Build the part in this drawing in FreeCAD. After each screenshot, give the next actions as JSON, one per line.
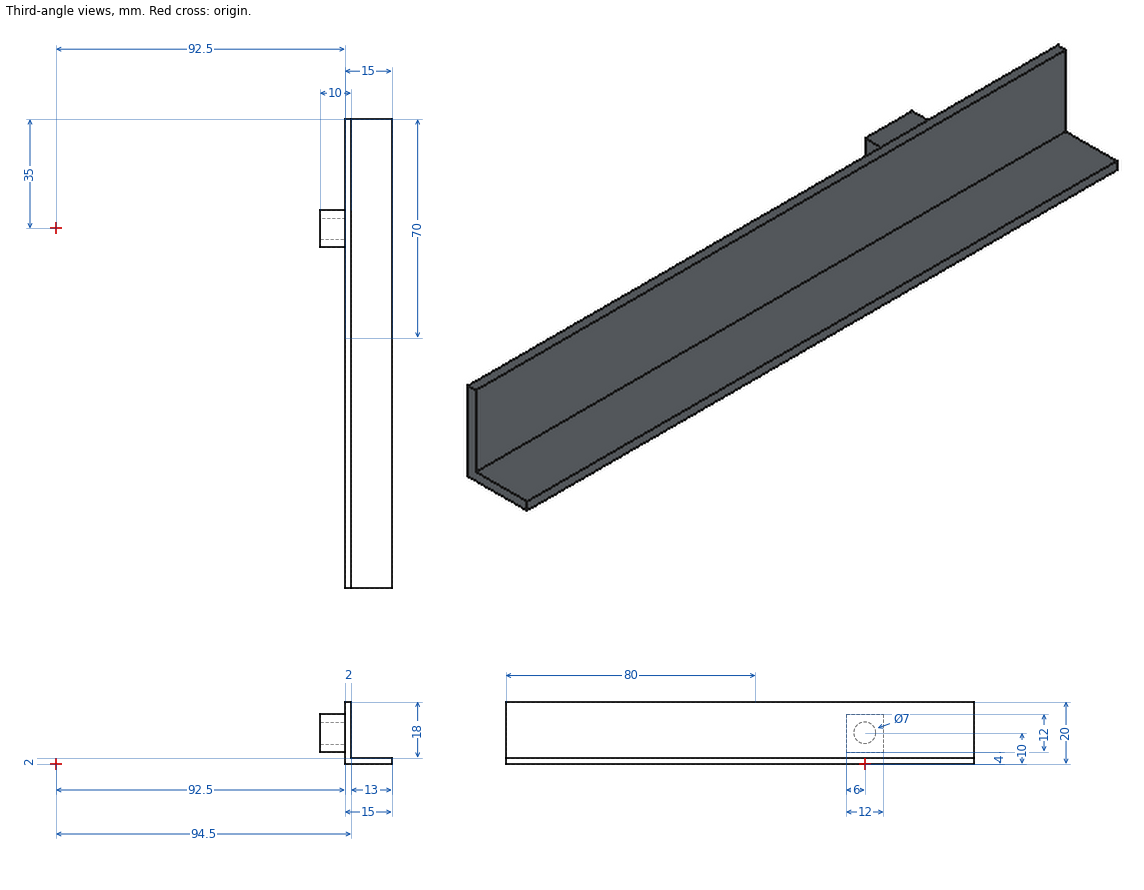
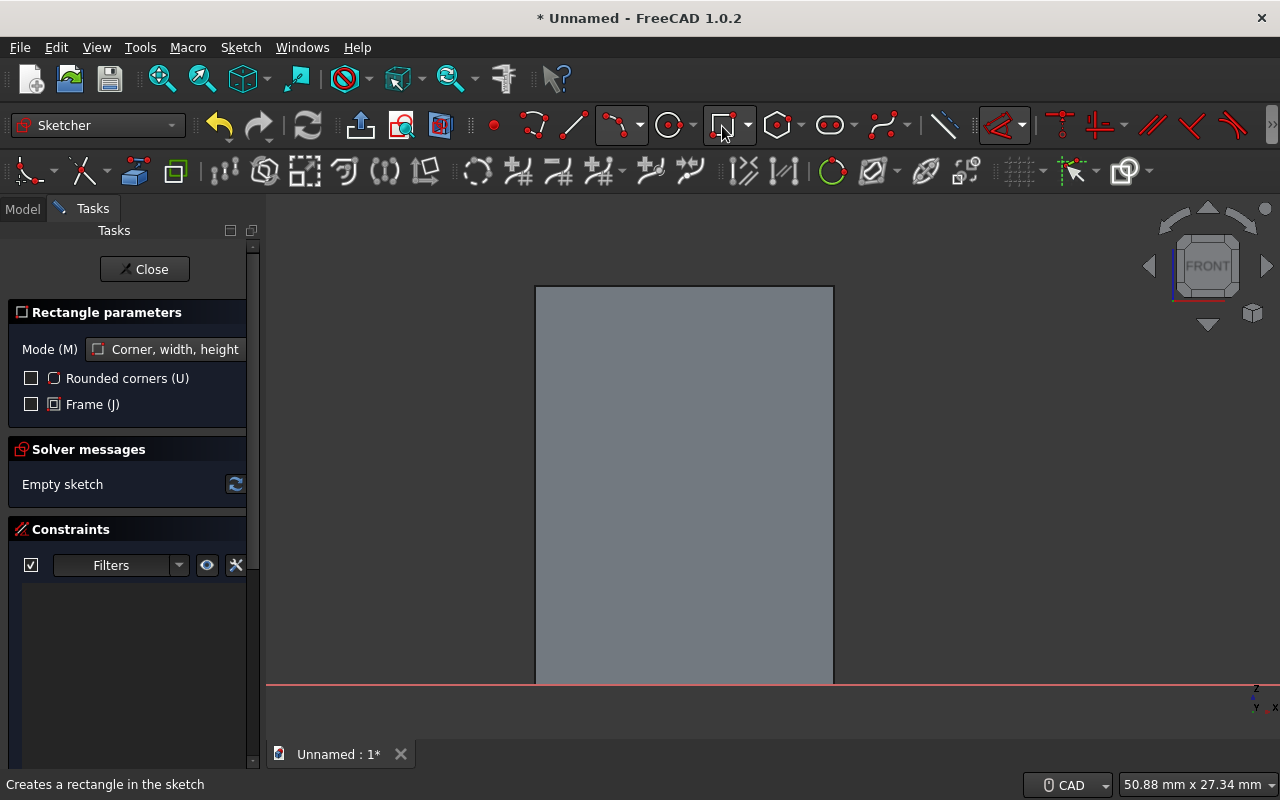
{"action": "left_click", "coordinate": [575, 286]}
{"action": "left_click", "coordinate": [834, 645]}
{"action": "key", "text": "Escape"}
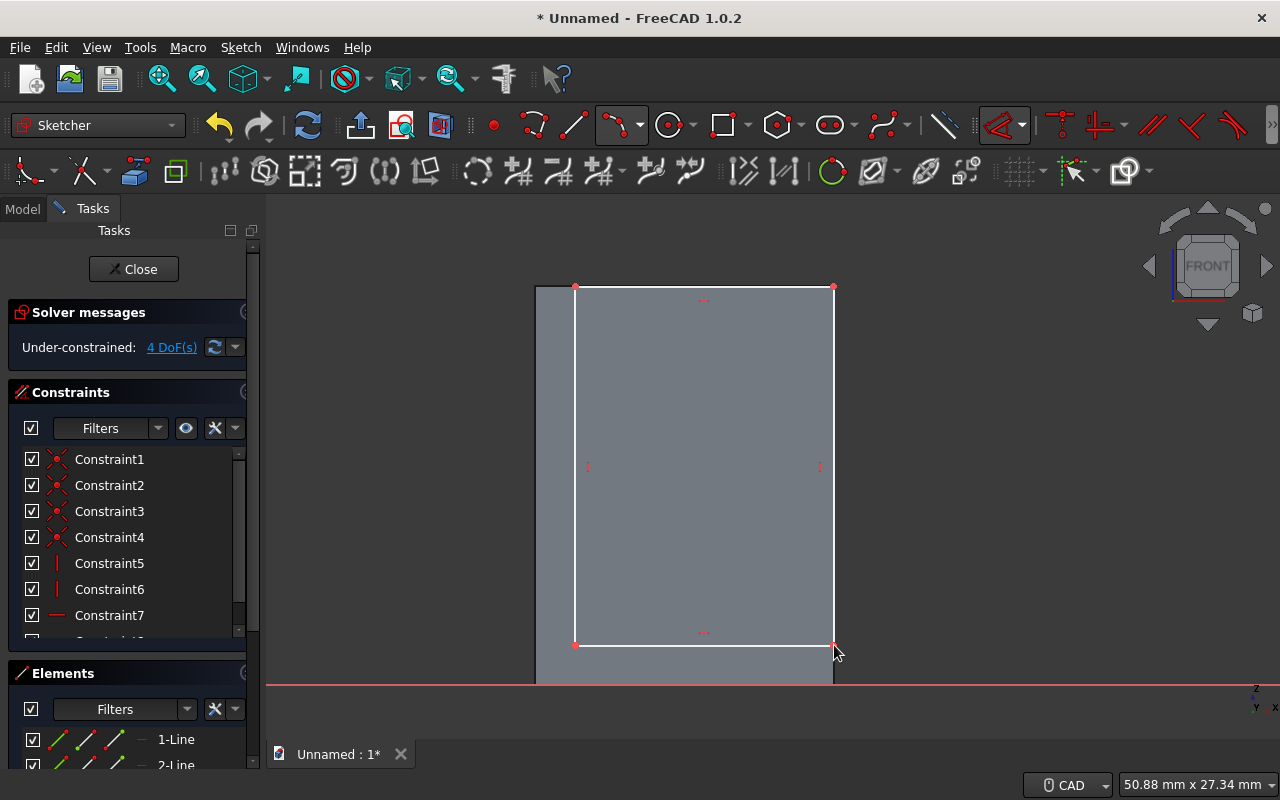
{"action": "left_click", "coordinate": [575, 395]}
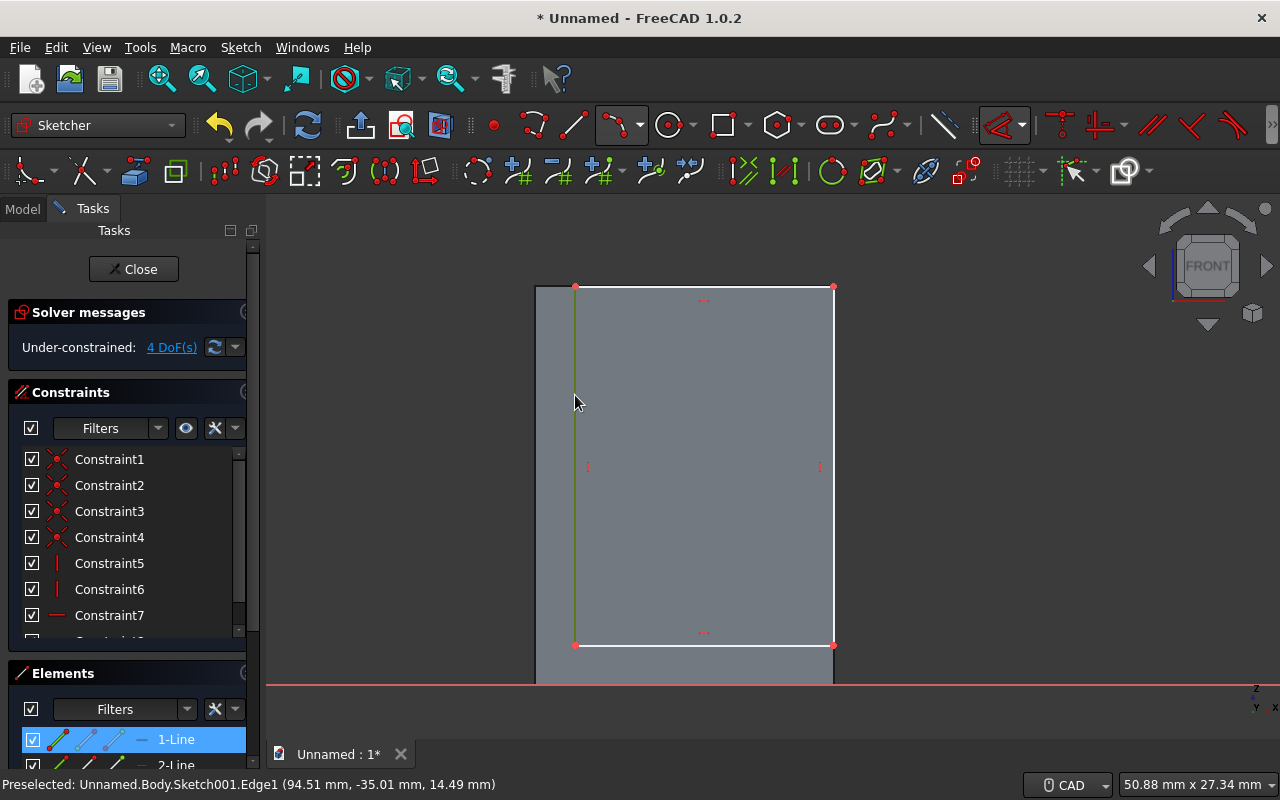
{"action": "key", "text": "i"}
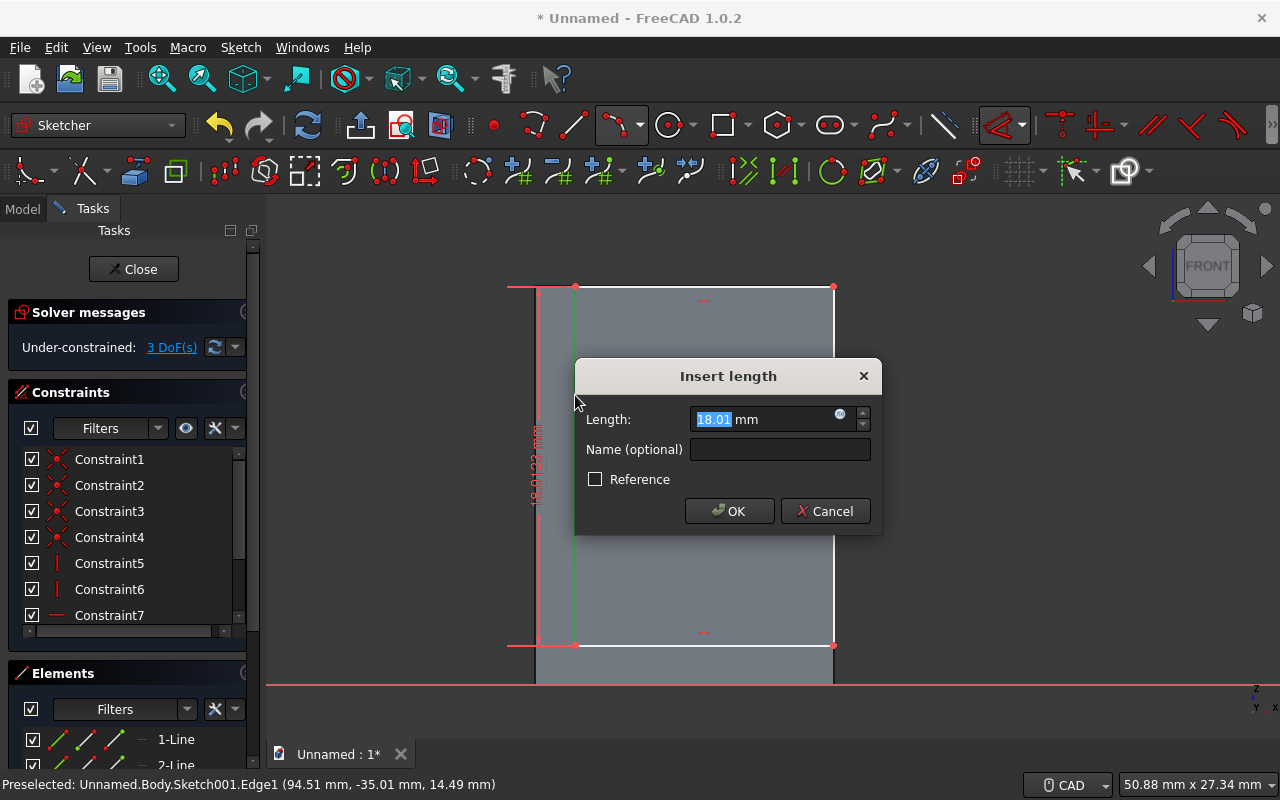
{"action": "type", "text": "18"}
{"action": "key", "text": "Return"}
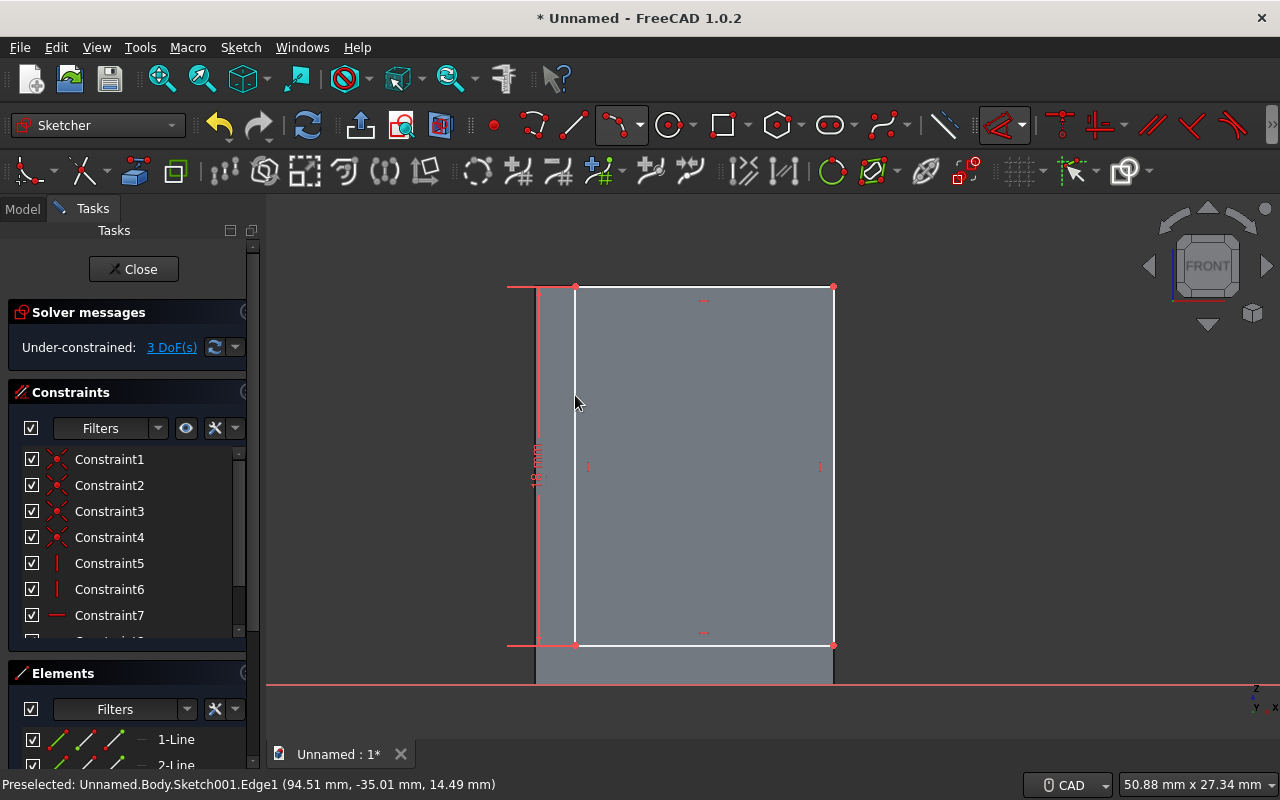
{"action": "left_click", "coordinate": [653, 646]}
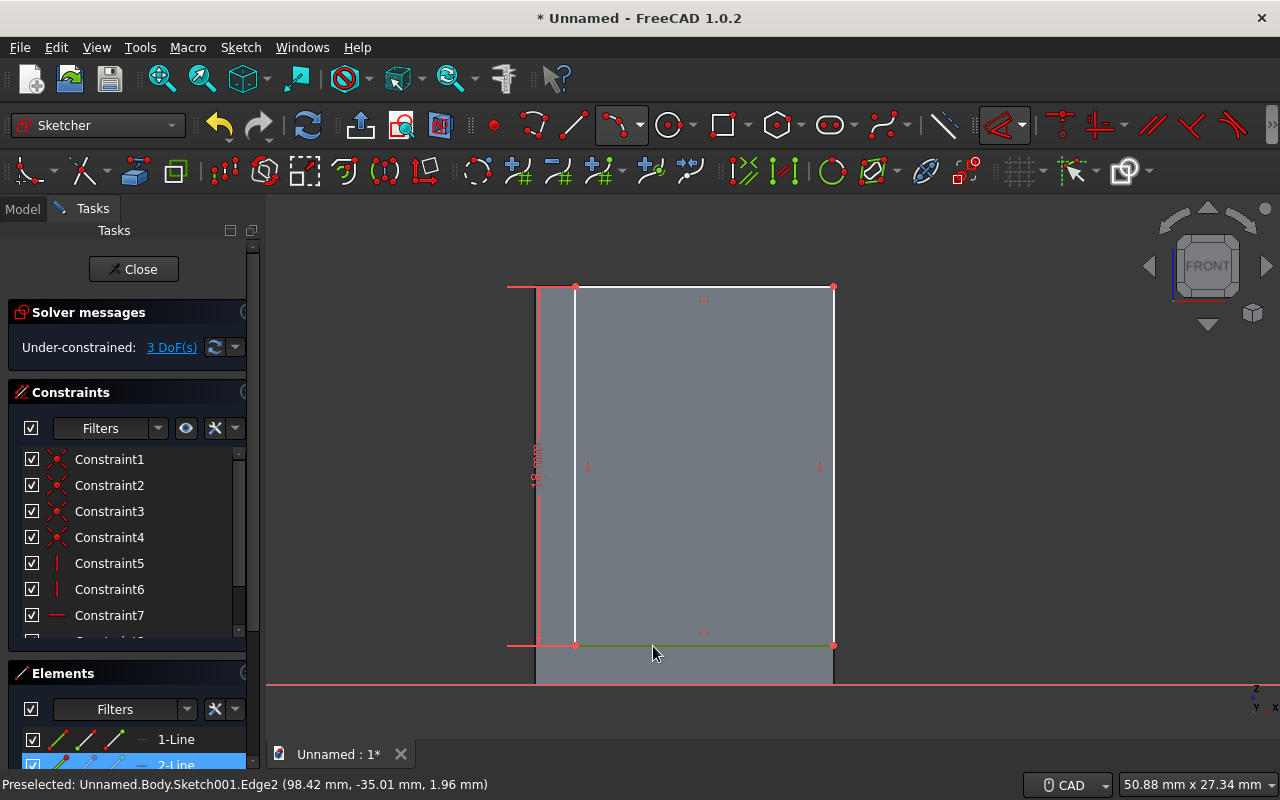
{"action": "left_click", "coordinate": [1024, 126]}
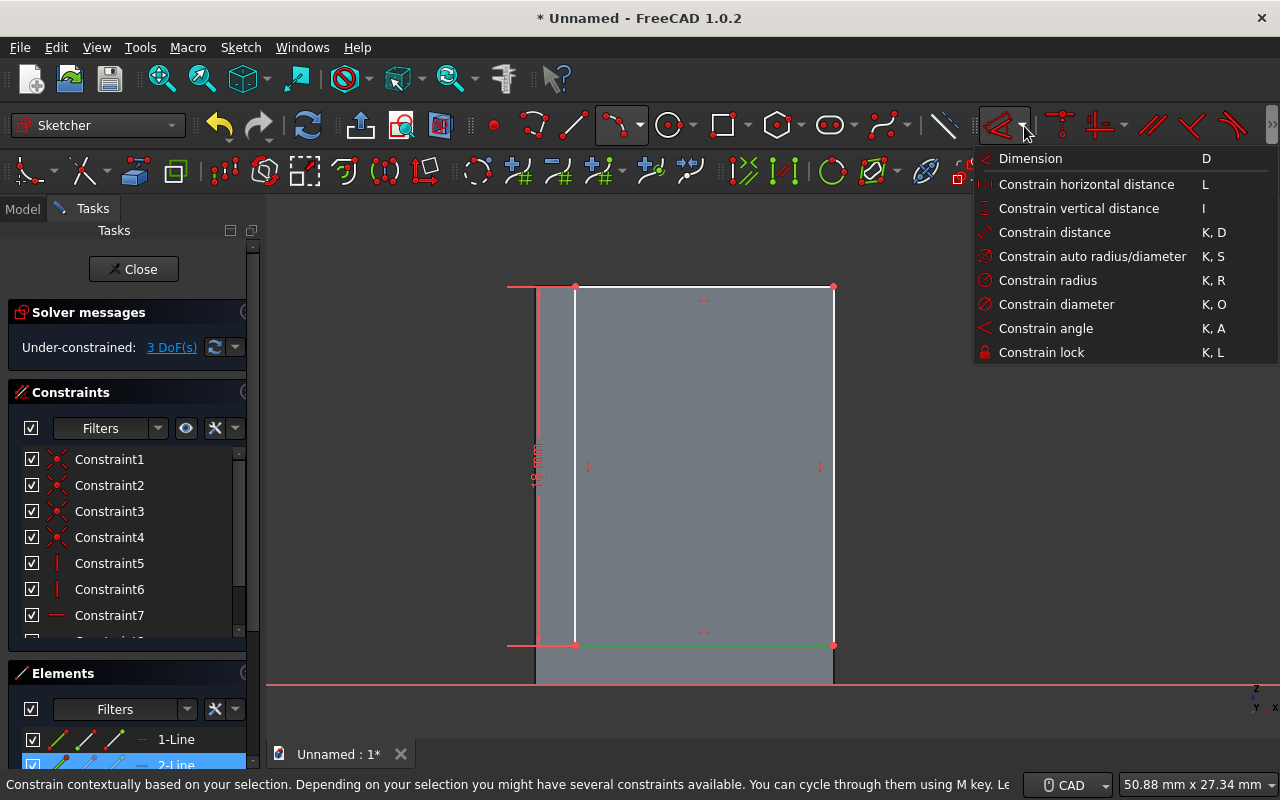
{"action": "left_click", "coordinate": [1126, 184]}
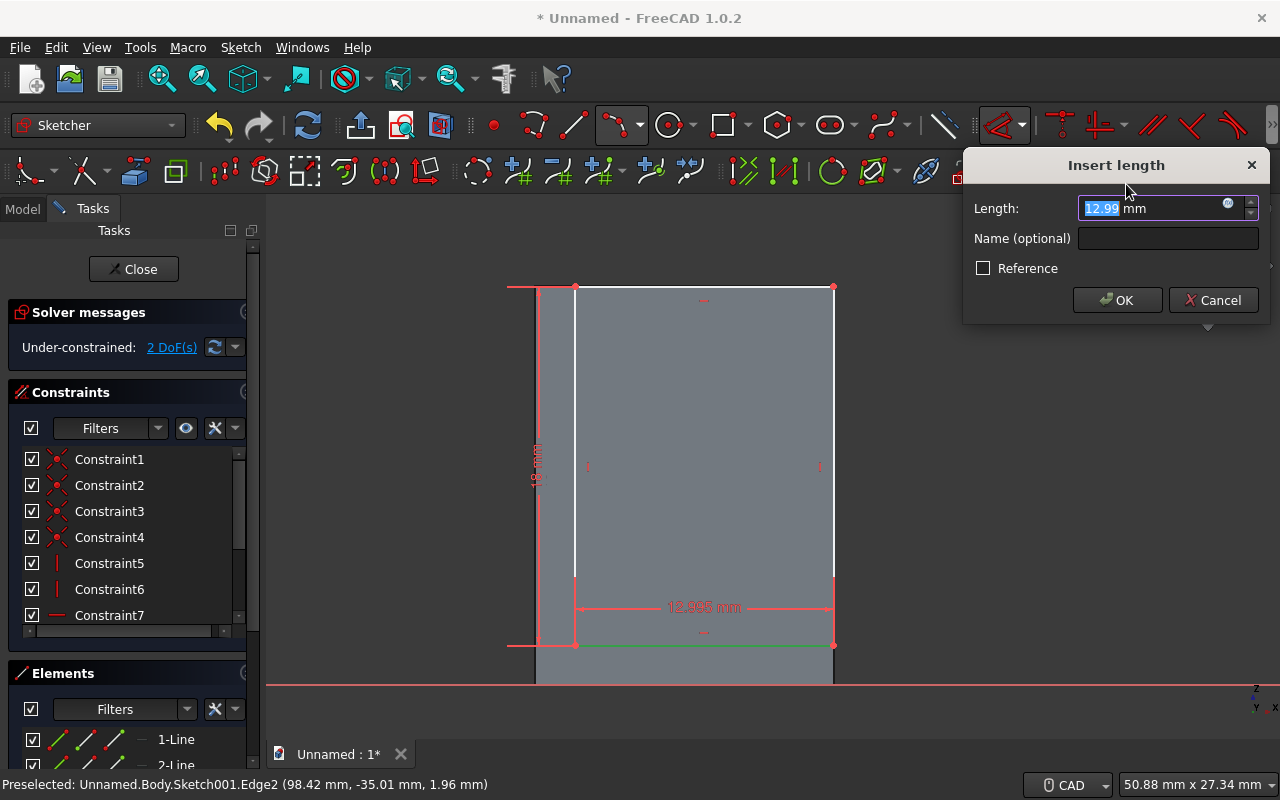
{"action": "type", "text": "13"}
{"action": "key", "text": "Return"}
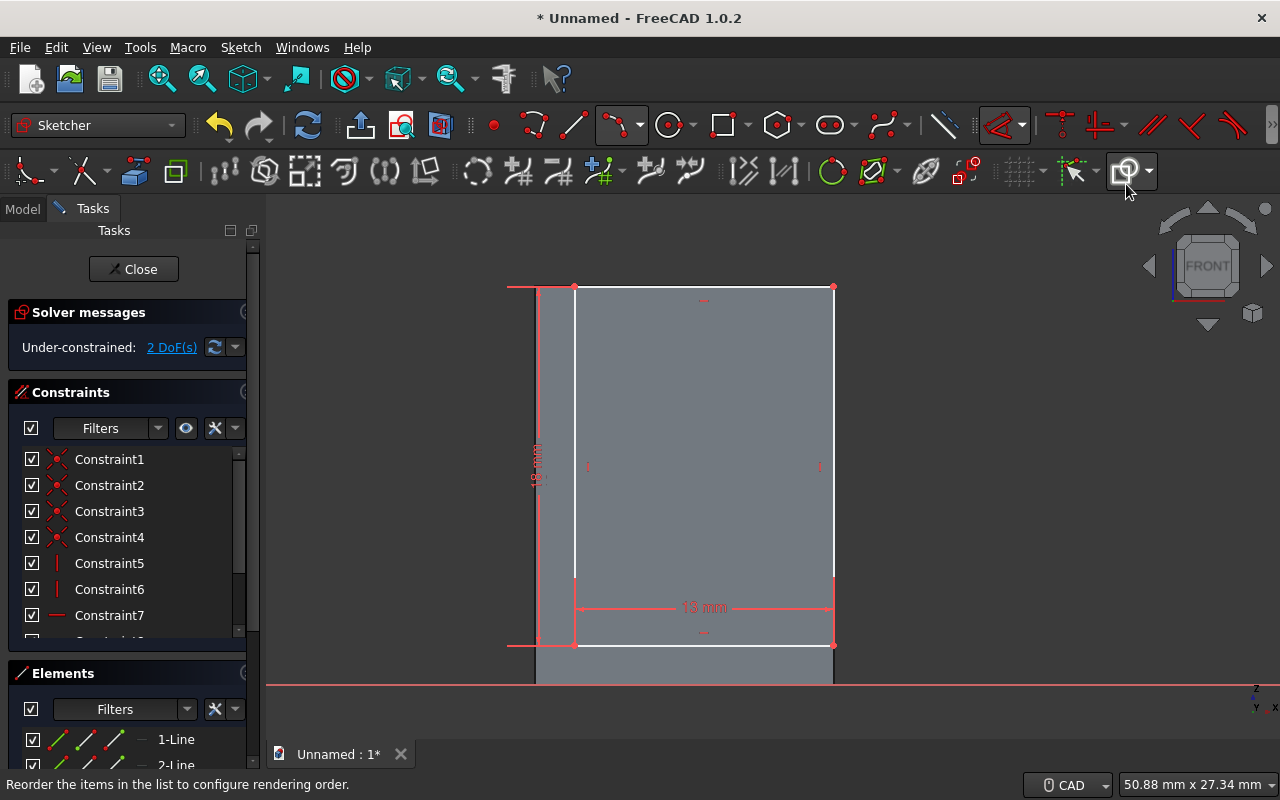
{"action": "left_click", "coordinate": [575, 646]}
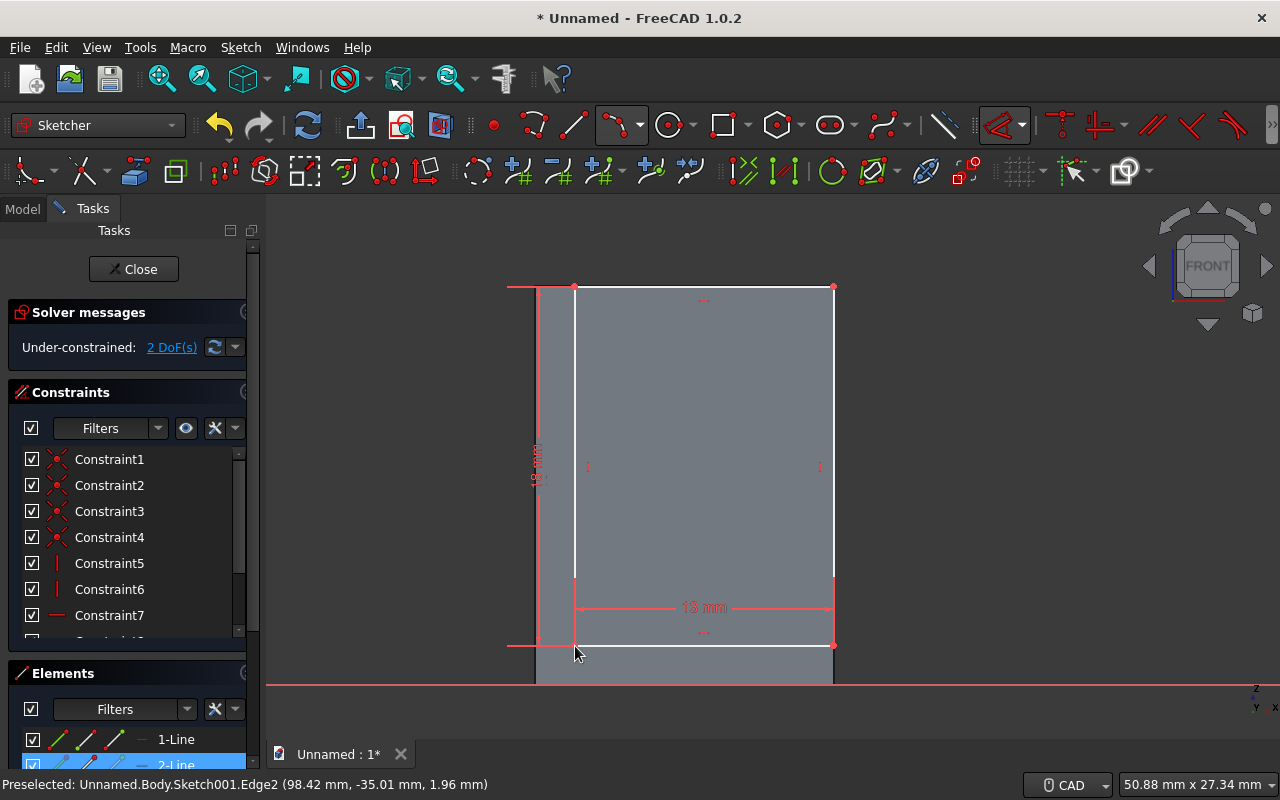
{"action": "left_click", "coordinate": [1024, 126]}